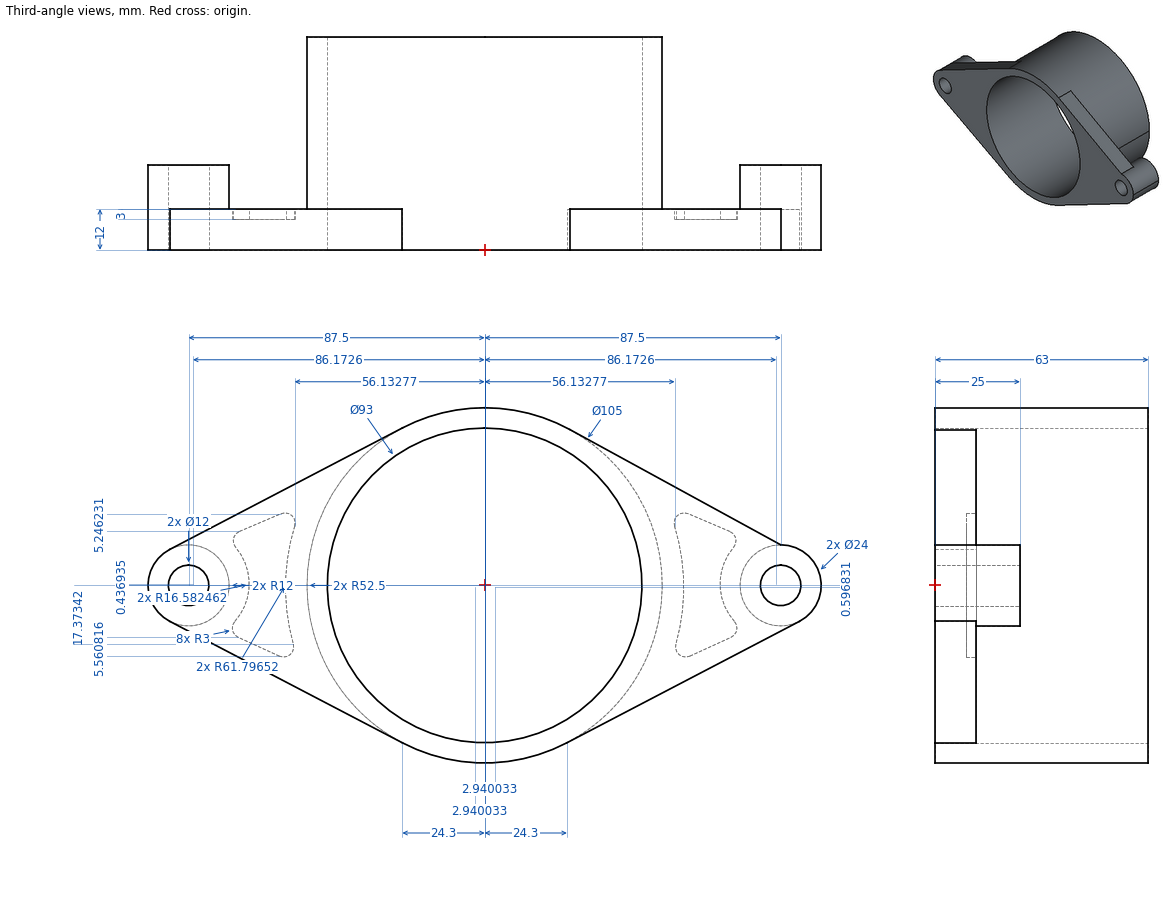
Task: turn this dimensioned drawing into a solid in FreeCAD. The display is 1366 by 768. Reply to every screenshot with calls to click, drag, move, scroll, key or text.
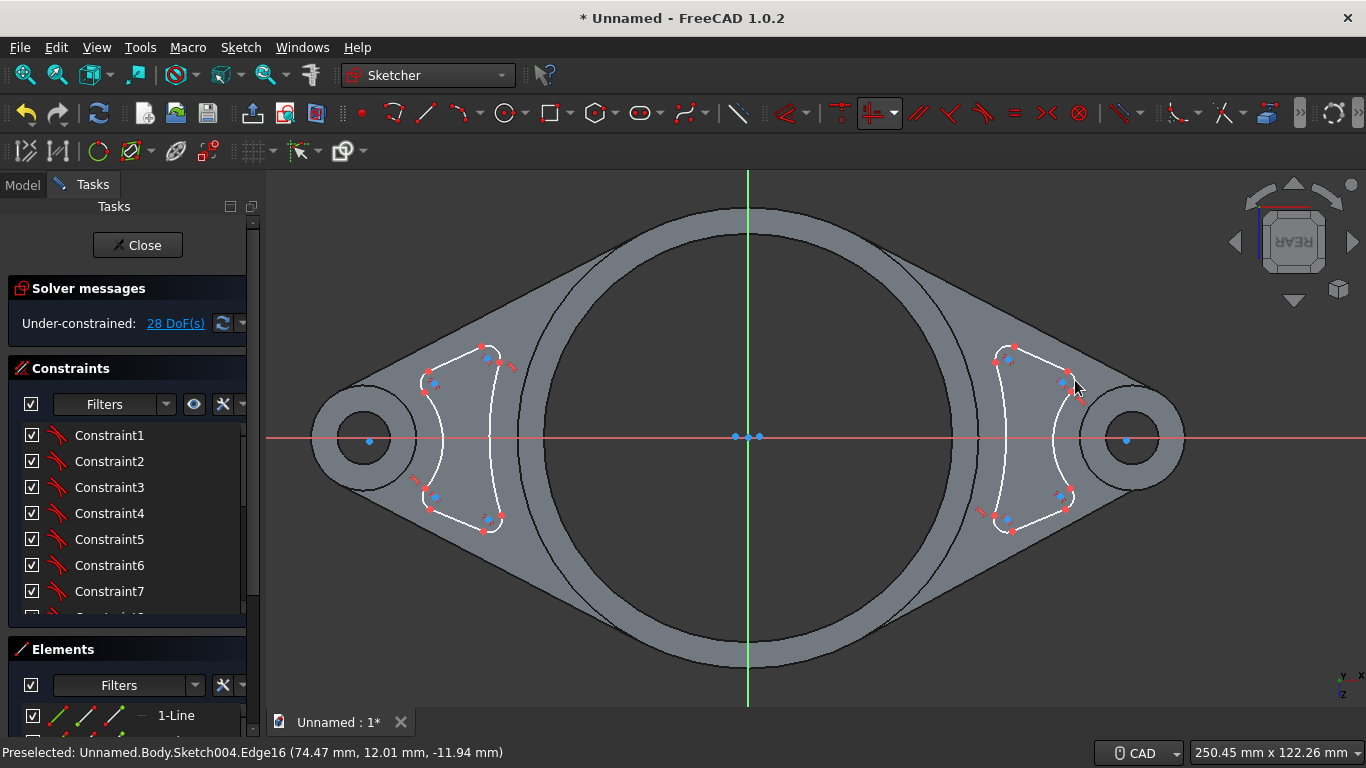
click(421, 381)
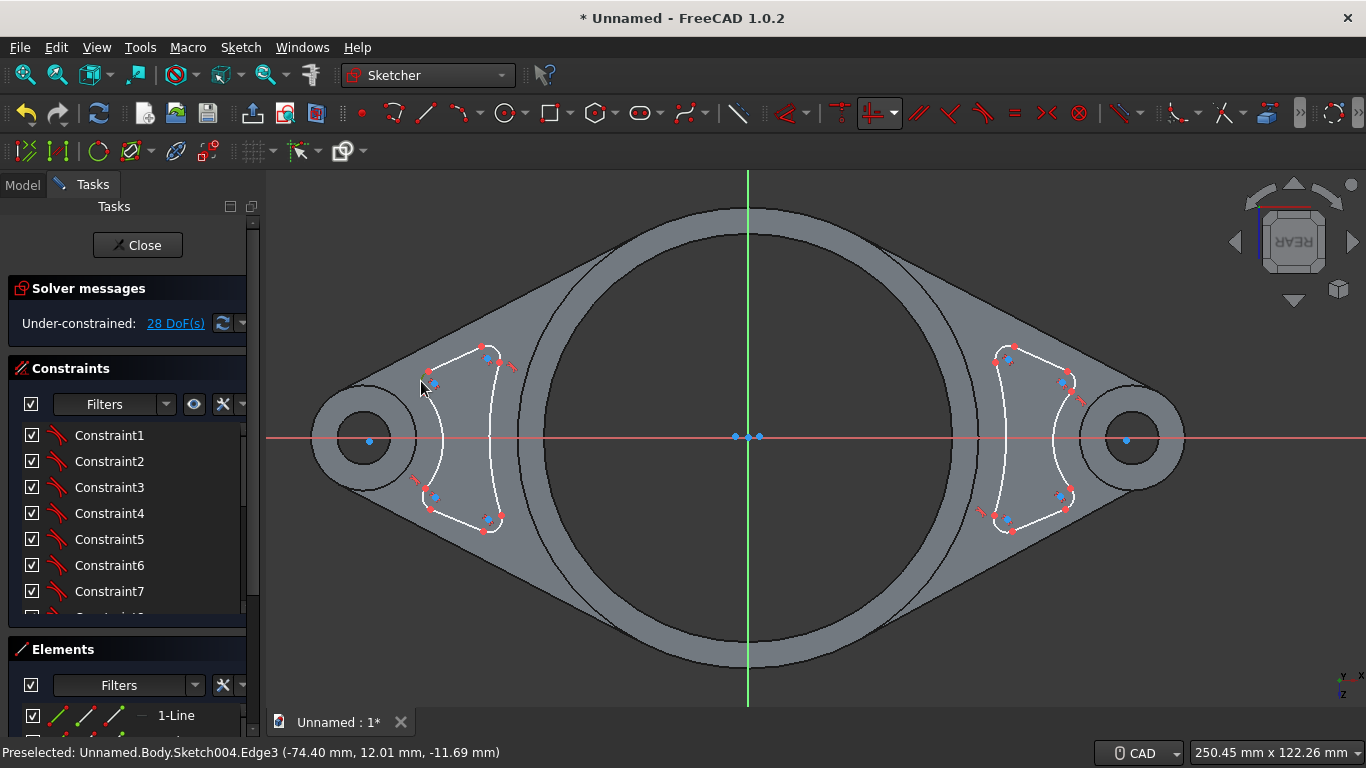
click(423, 500)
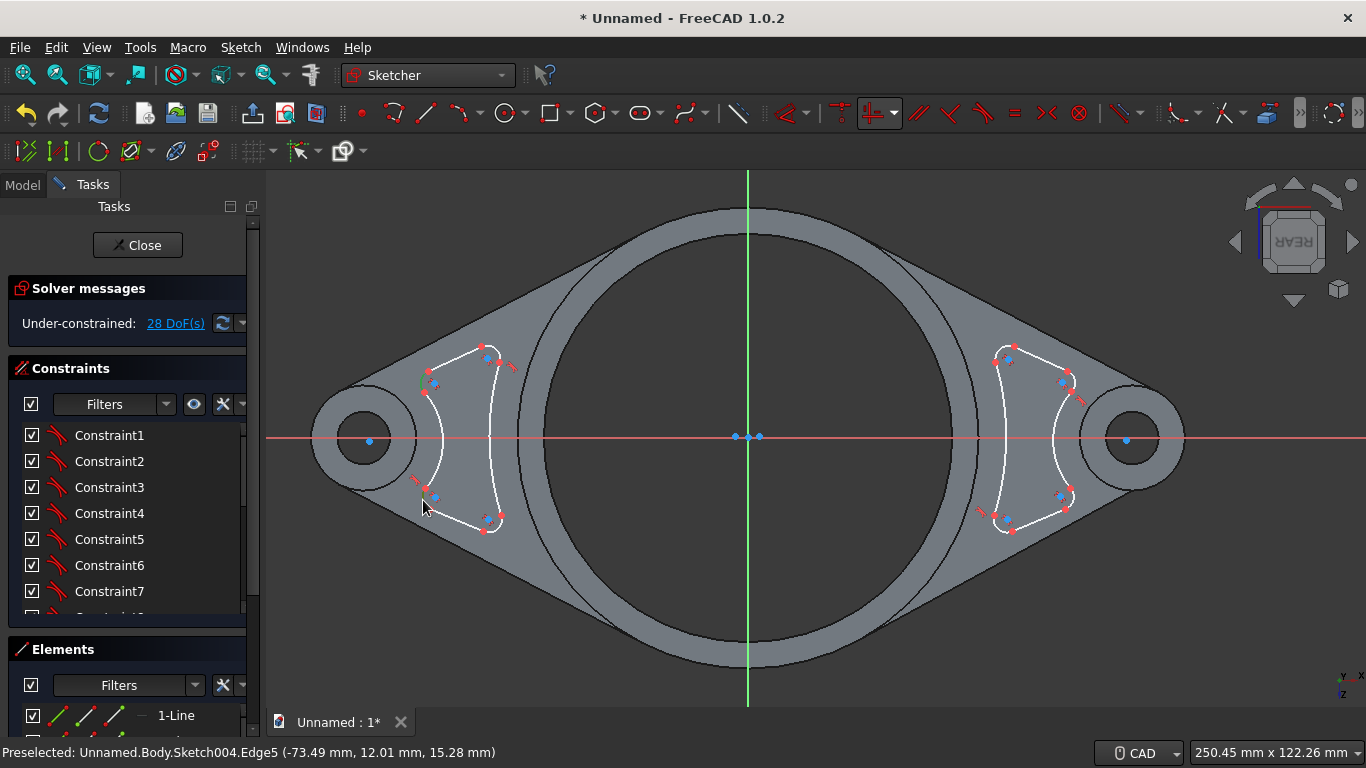
click(498, 529)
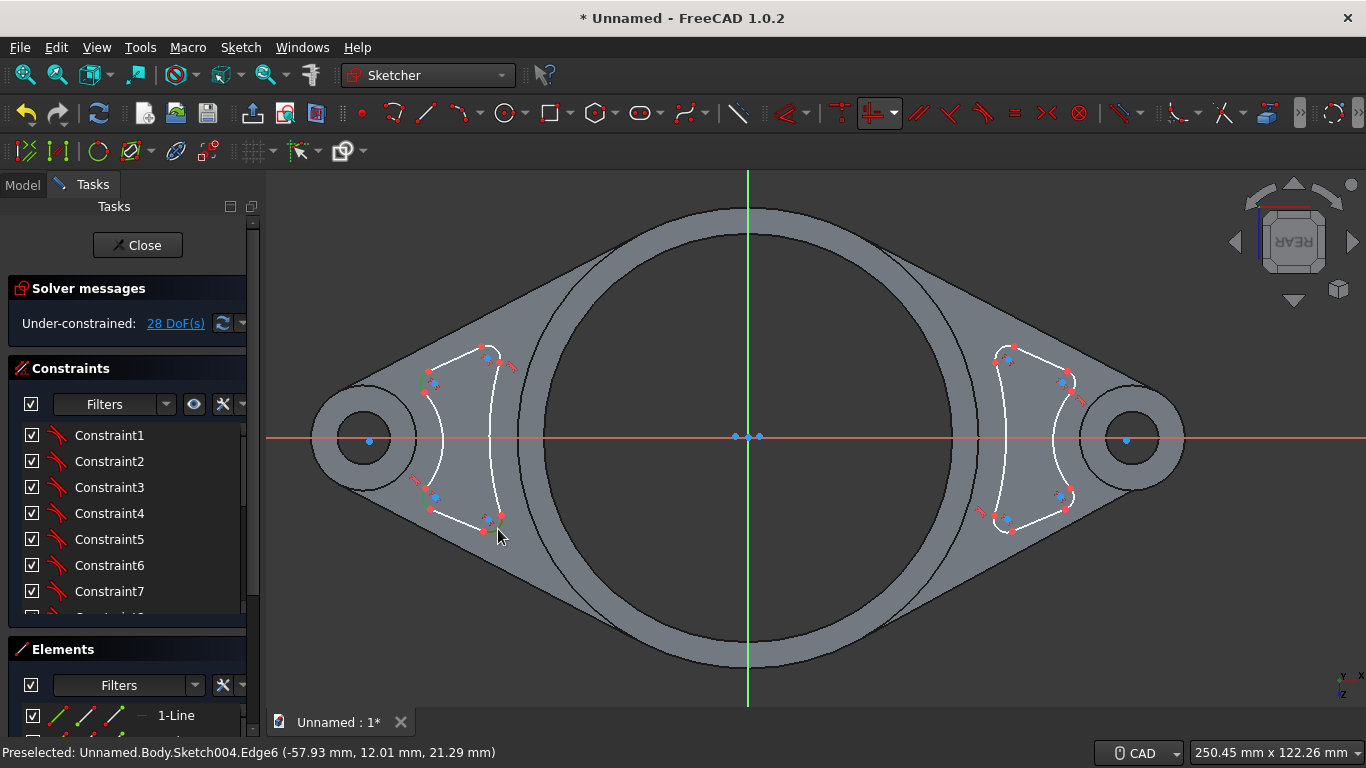
click(496, 349)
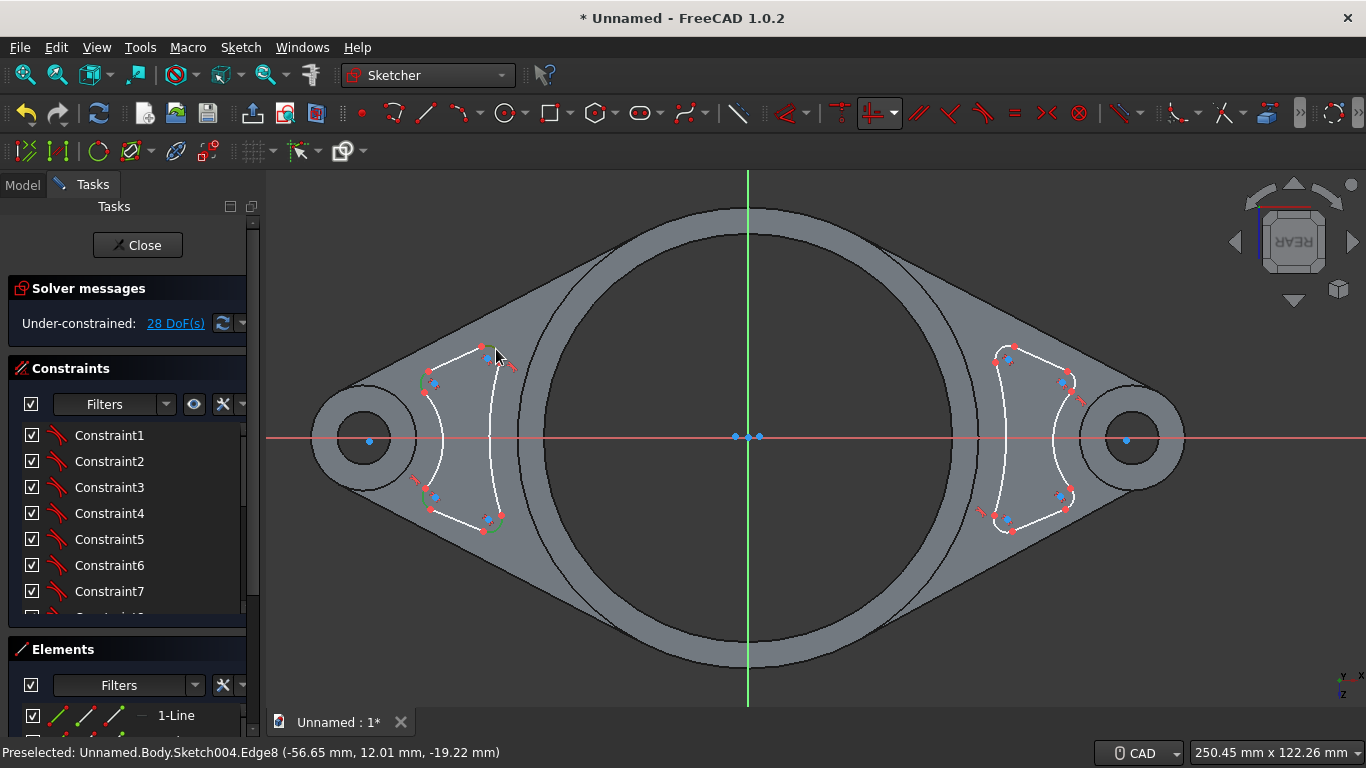
click(1000, 349)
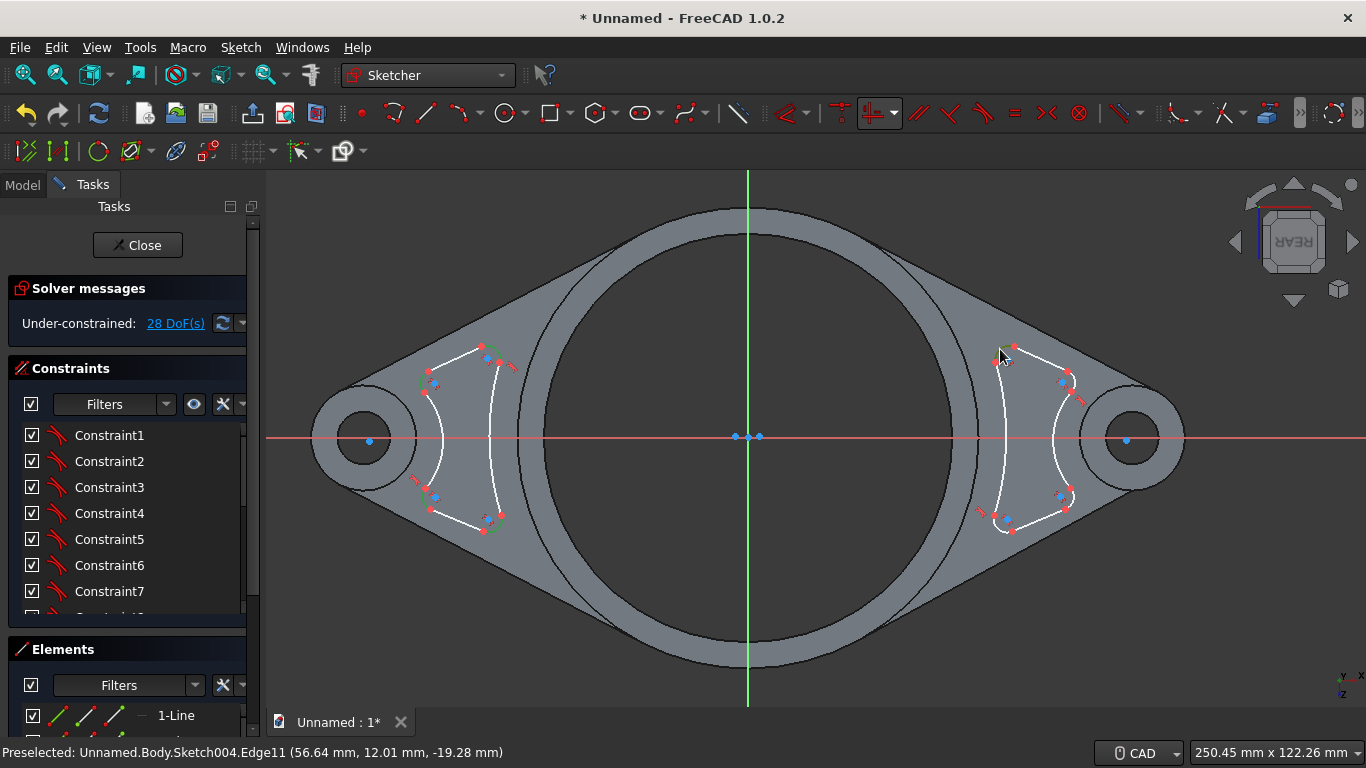
click(998, 529)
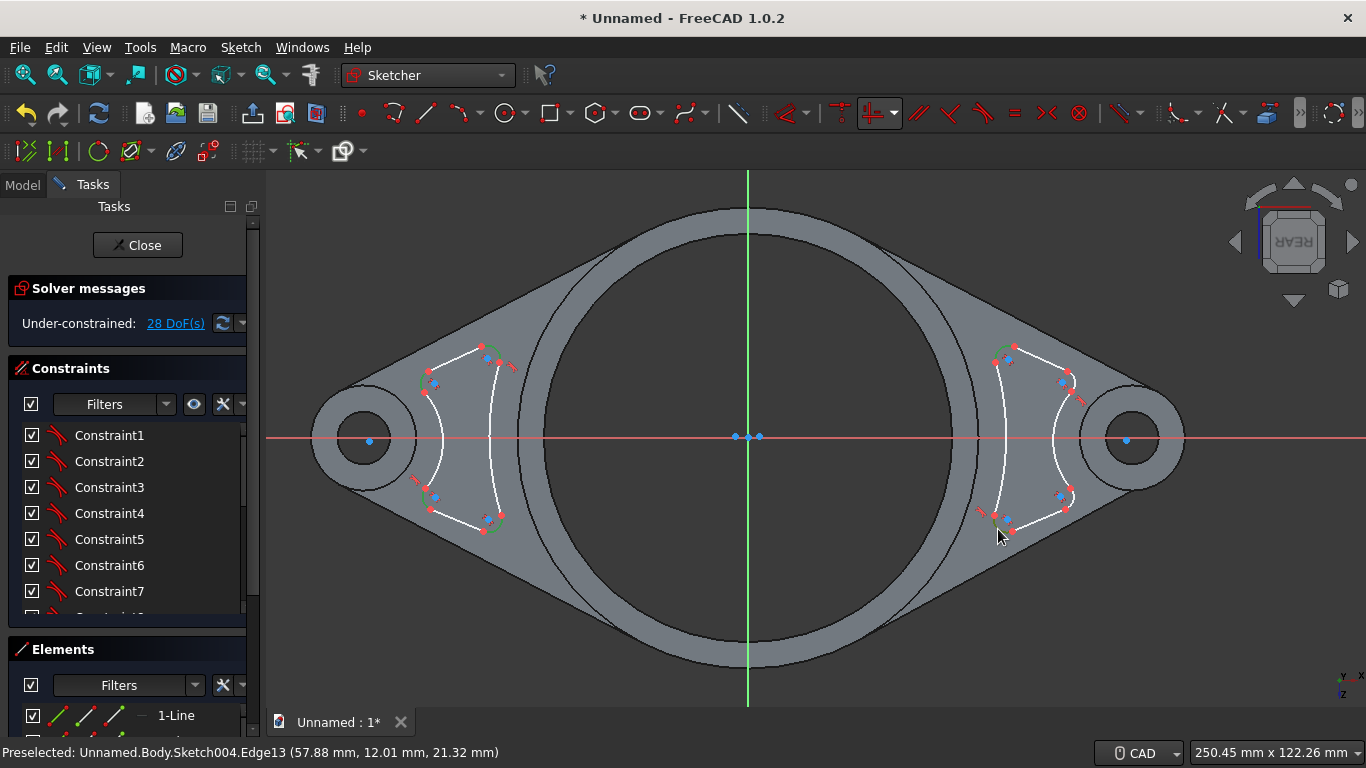
click(1073, 500)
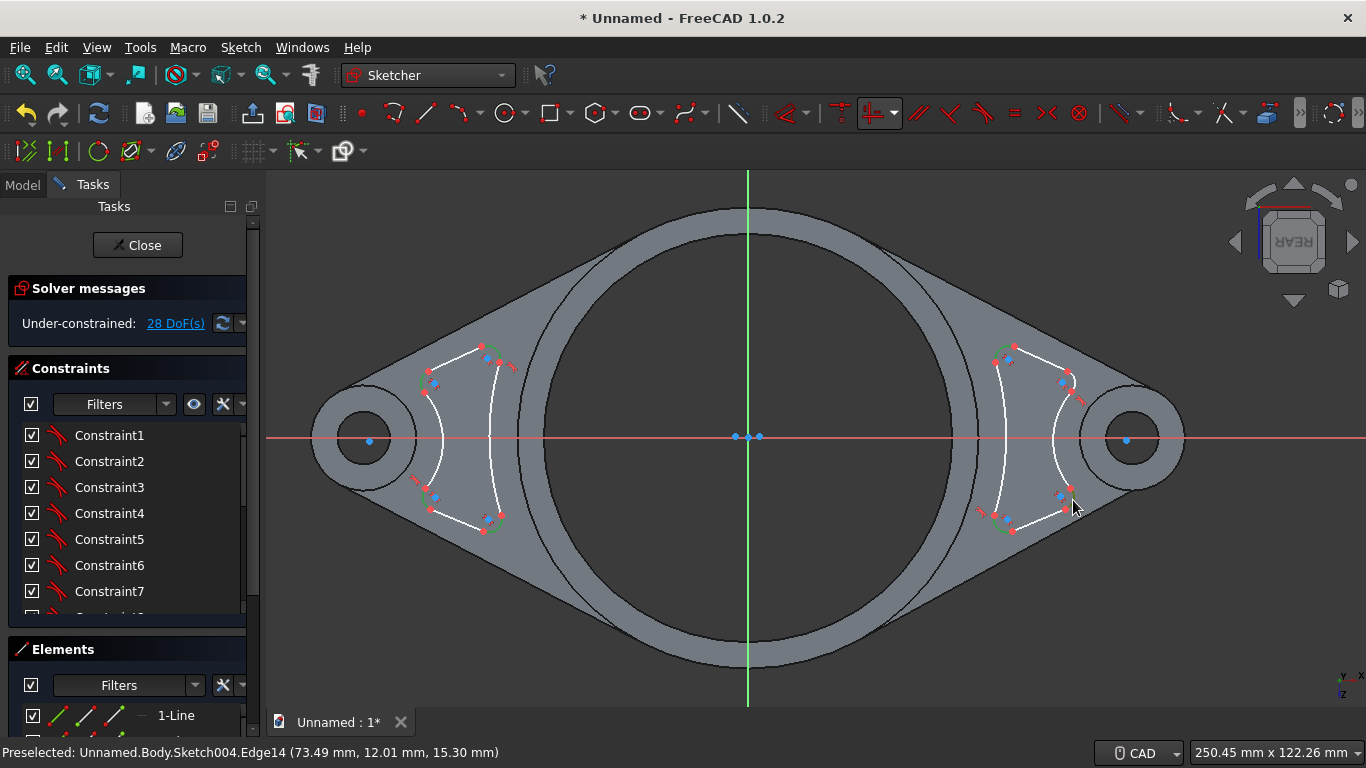
click(1075, 380)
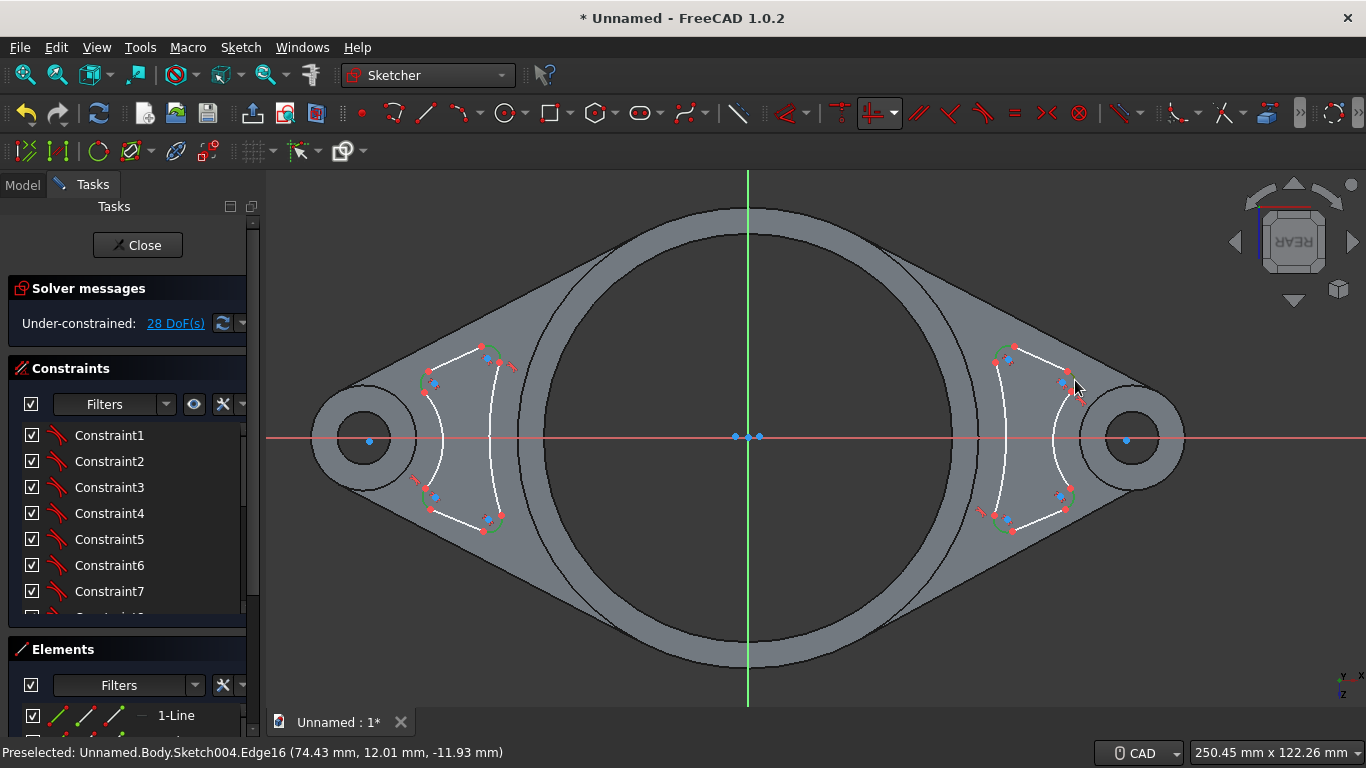
key(e)